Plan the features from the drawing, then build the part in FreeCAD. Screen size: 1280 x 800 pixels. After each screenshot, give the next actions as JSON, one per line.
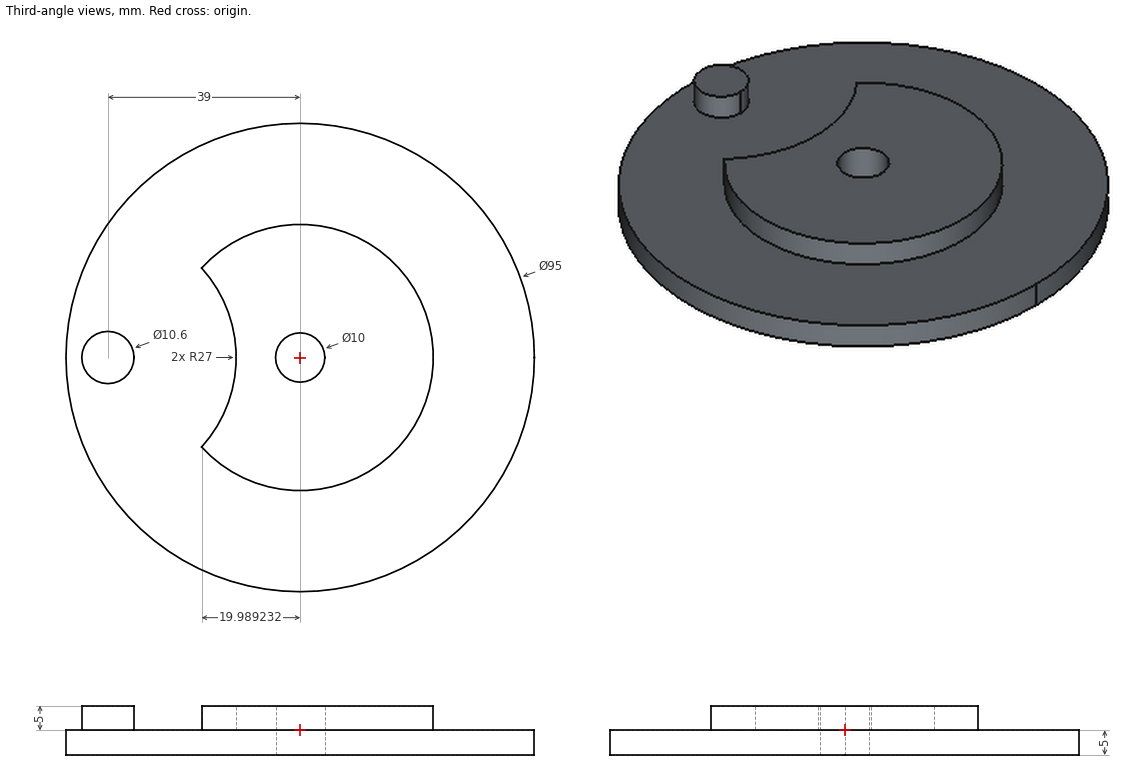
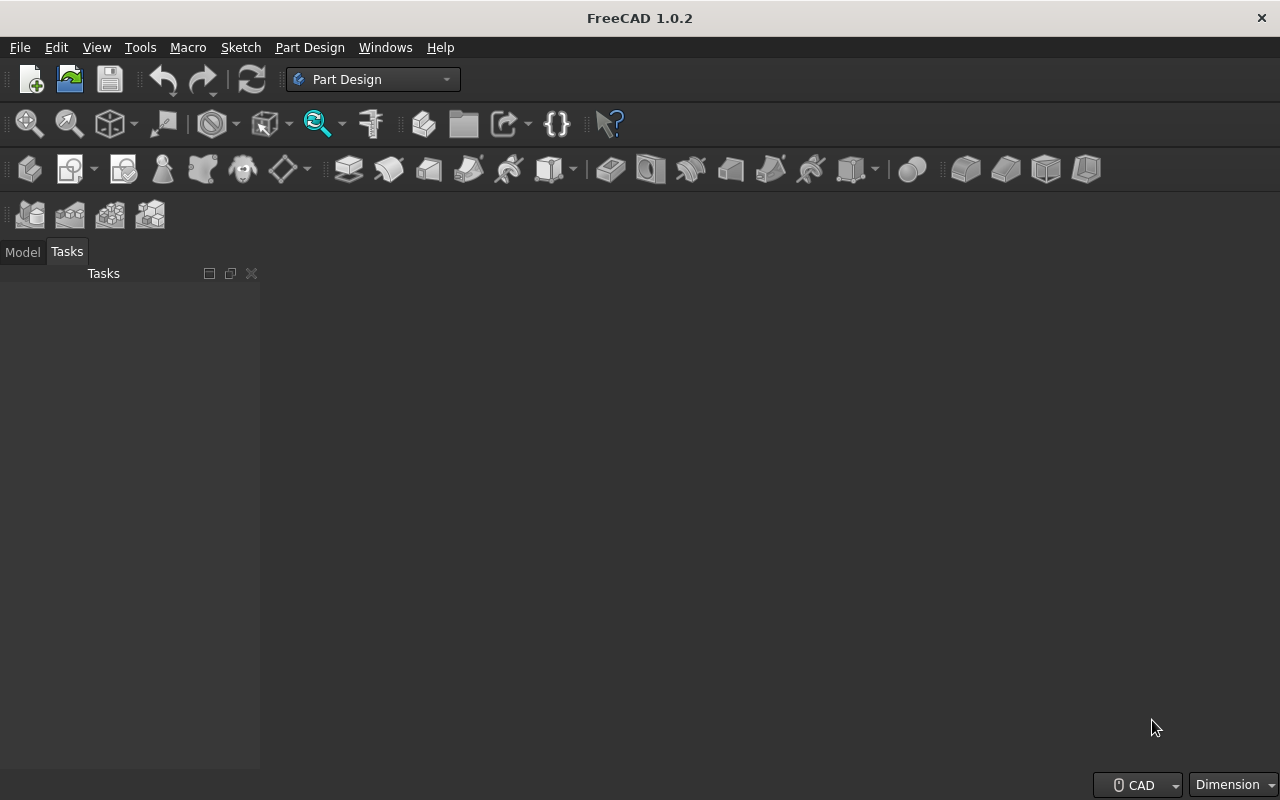
{"action": "key", "text": "ctrl+n"}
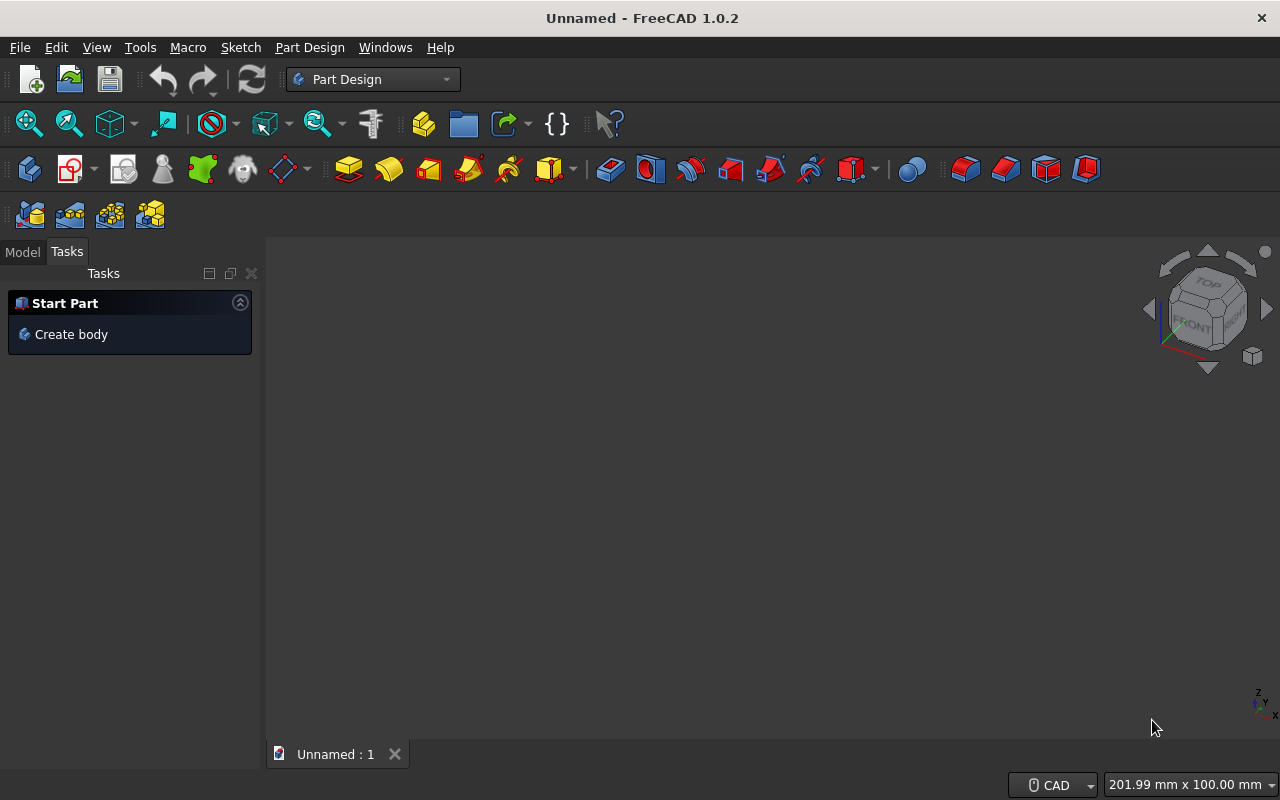
{"action": "left_click", "coordinate": [70, 170]}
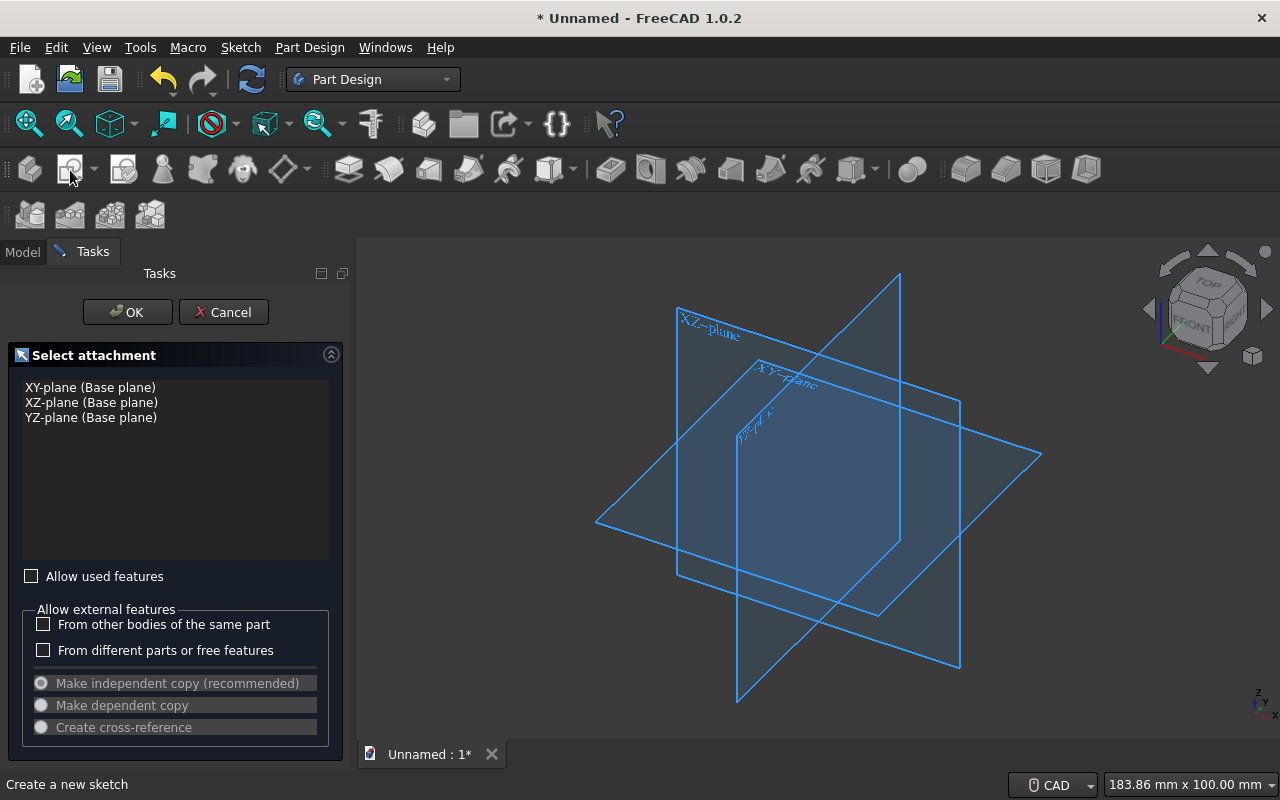
{"action": "left_click", "coordinate": [82, 388]}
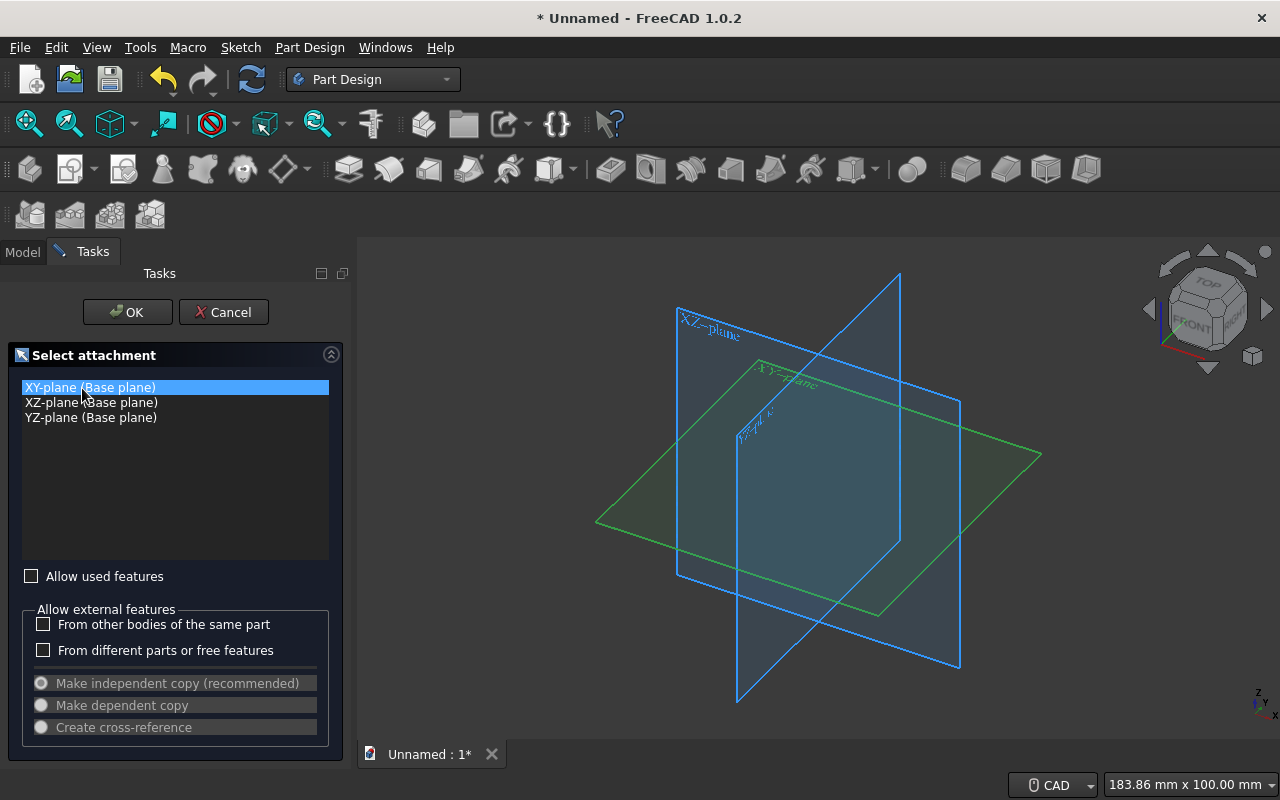
{"action": "left_click", "coordinate": [128, 312]}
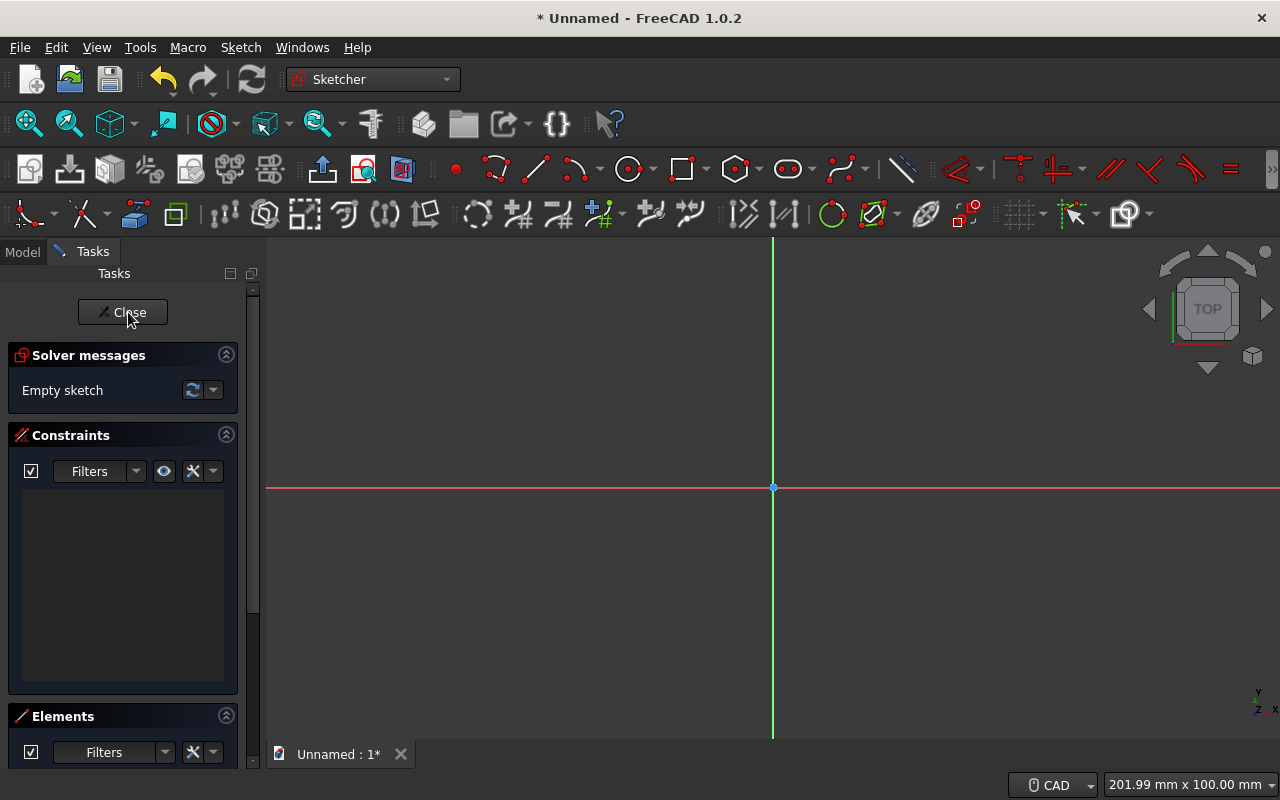
{"action": "scroll", "coordinate": [565, 488], "scroll_direction": "down", "scroll_amount": 2}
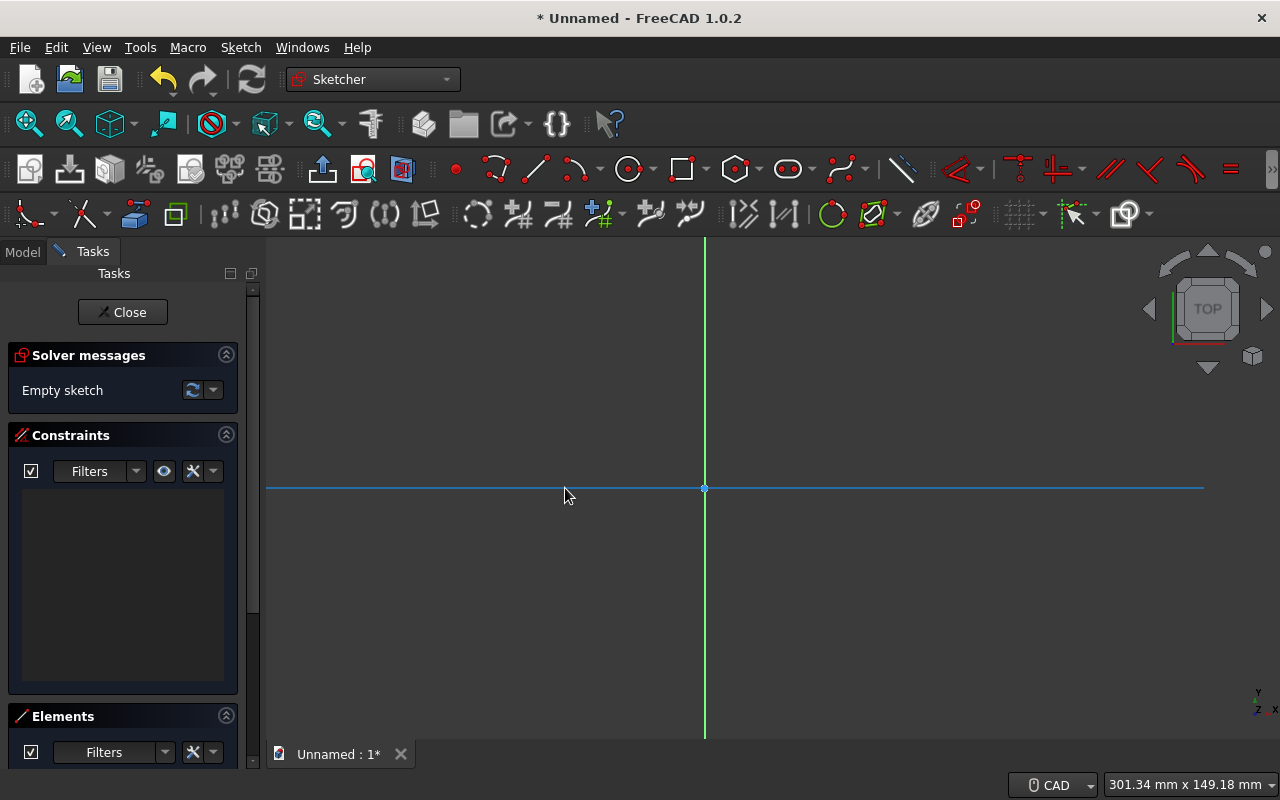
{"action": "left_click", "coordinate": [630, 170]}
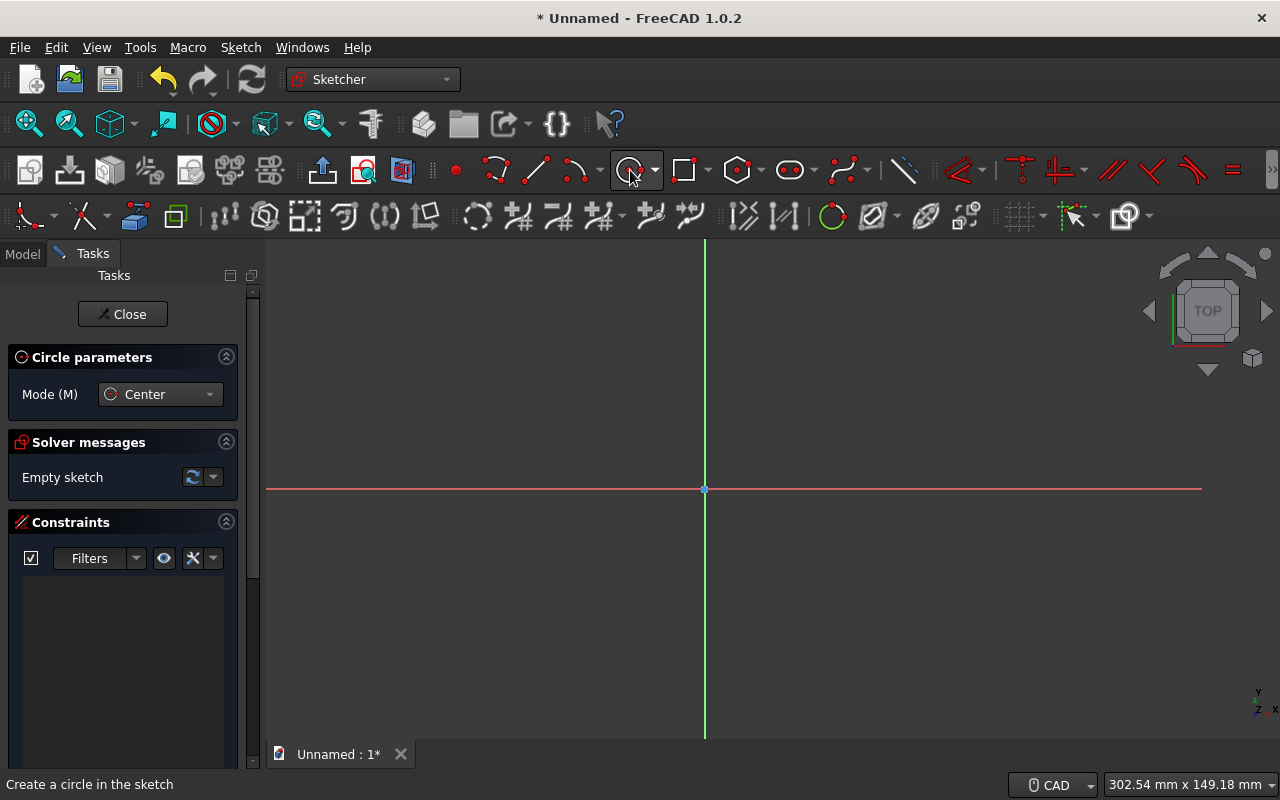
{"action": "left_click", "coordinate": [705, 489]}
{"action": "left_click", "coordinate": [817, 377]}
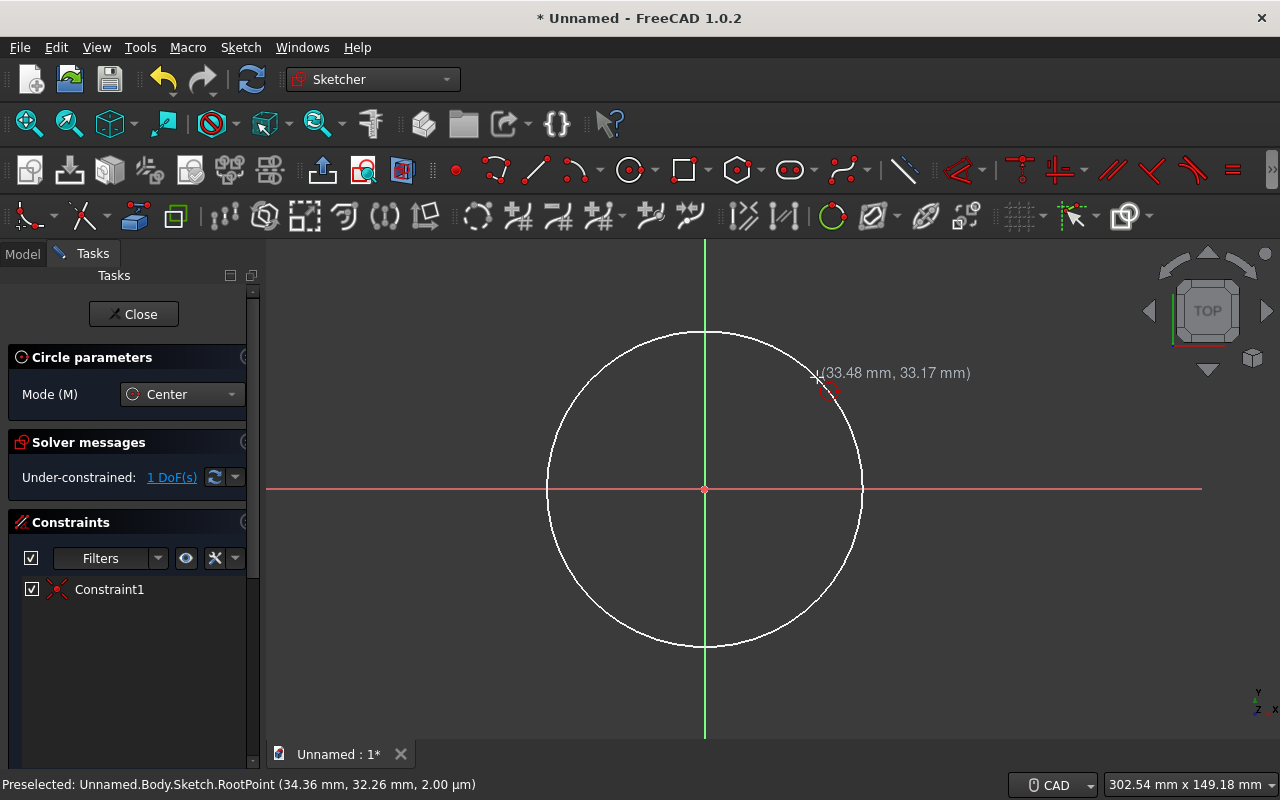
{"action": "scroll", "coordinate": [705, 489], "scroll_direction": "up", "scroll_amount": 2}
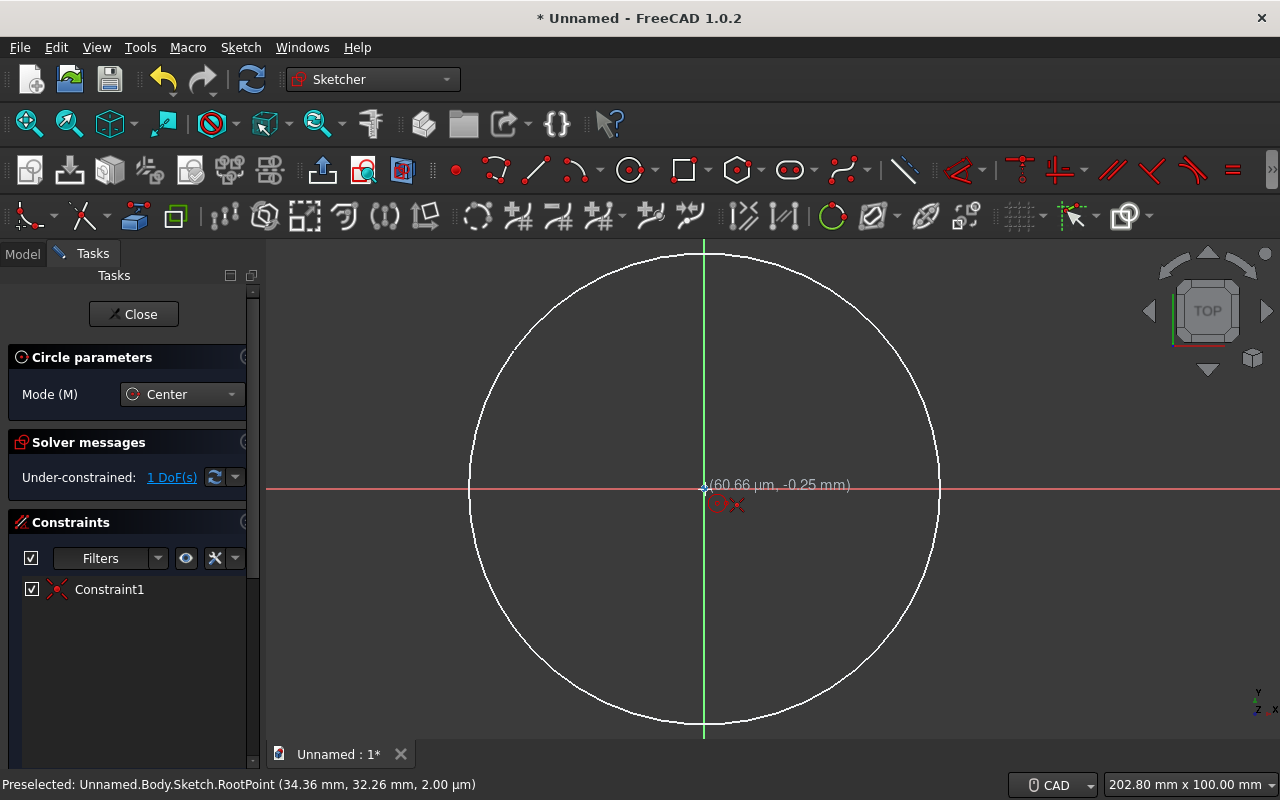
{"action": "left_click", "coordinate": [704, 489]}
{"action": "left_click", "coordinate": [722, 471]}
{"action": "key", "text": "Escape"}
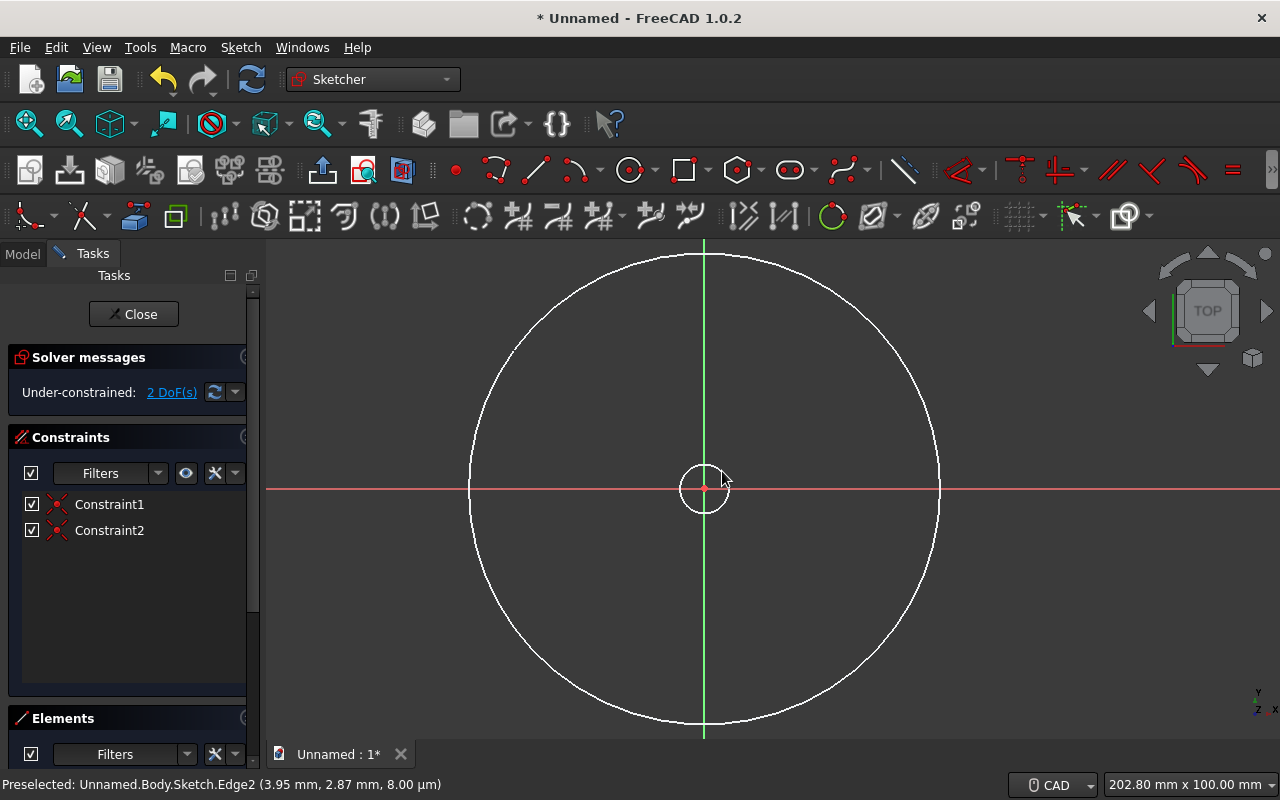
{"action": "left_click", "coordinate": [871, 322]}